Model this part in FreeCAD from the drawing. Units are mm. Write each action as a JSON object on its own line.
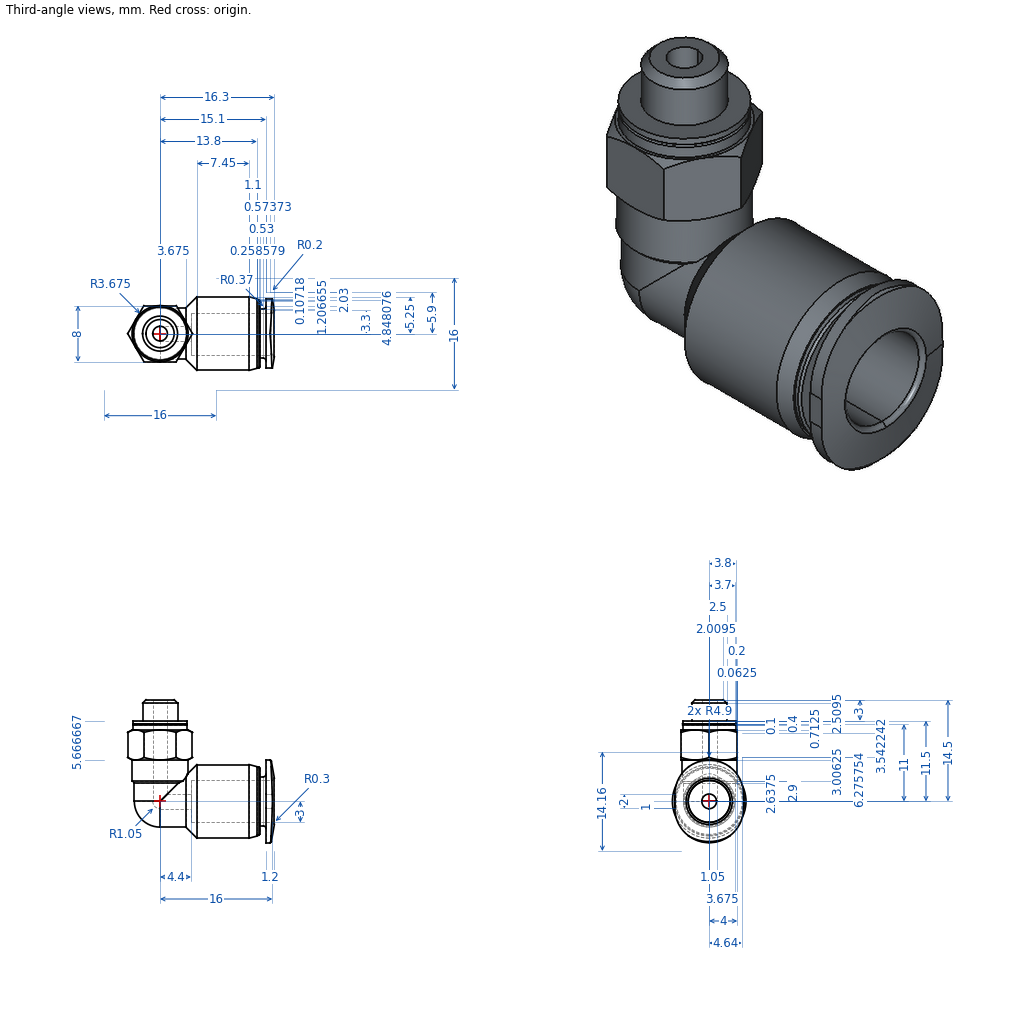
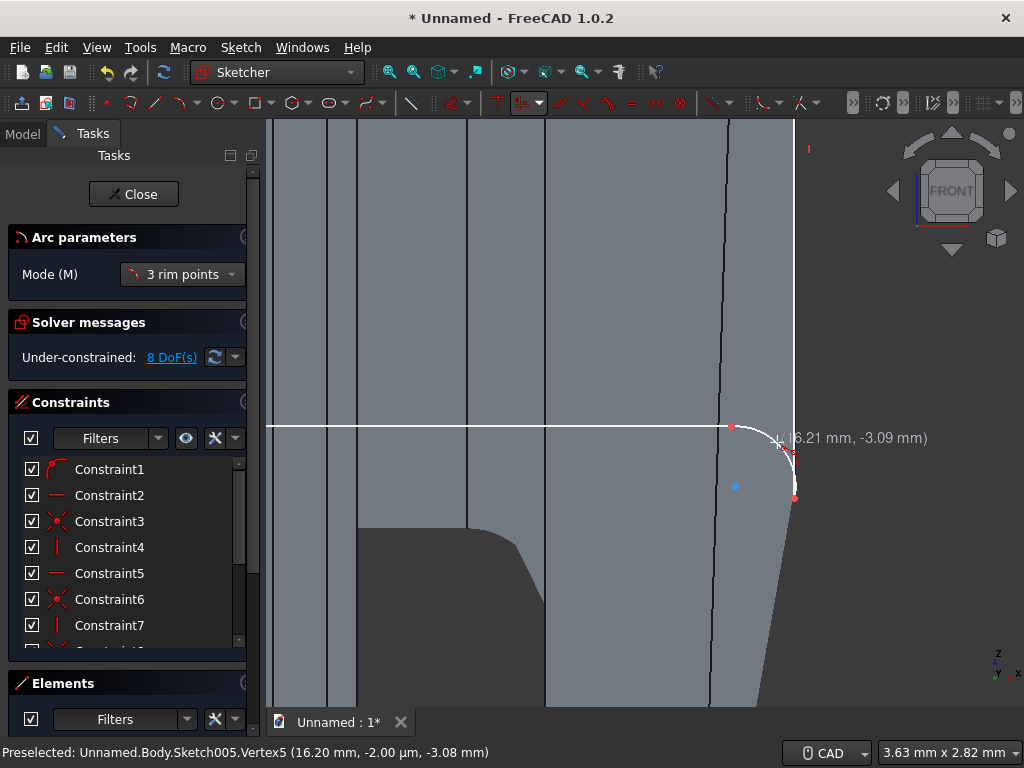
{"action": "scroll", "coordinate": [775, 447], "scroll_direction": "down", "scroll_amount": 11}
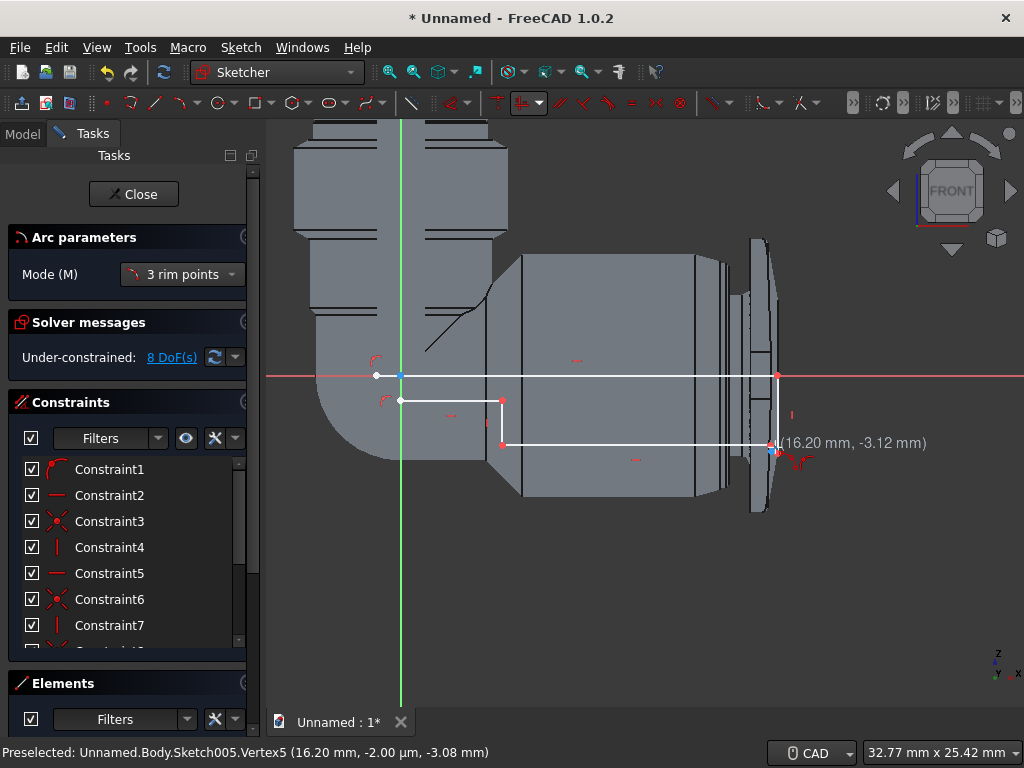
{"action": "left_click", "coordinate": [401, 401]}
{"action": "left_click", "coordinate": [377, 376]}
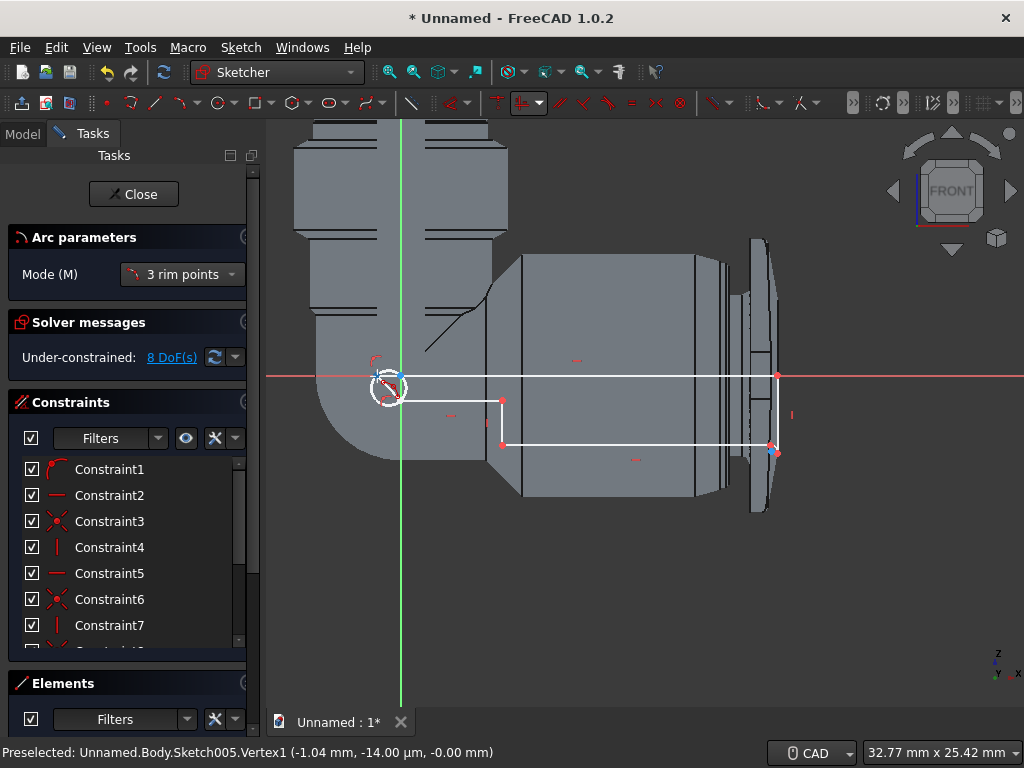
{"action": "scroll", "coordinate": [384, 393], "scroll_direction": "up", "scroll_amount": 5}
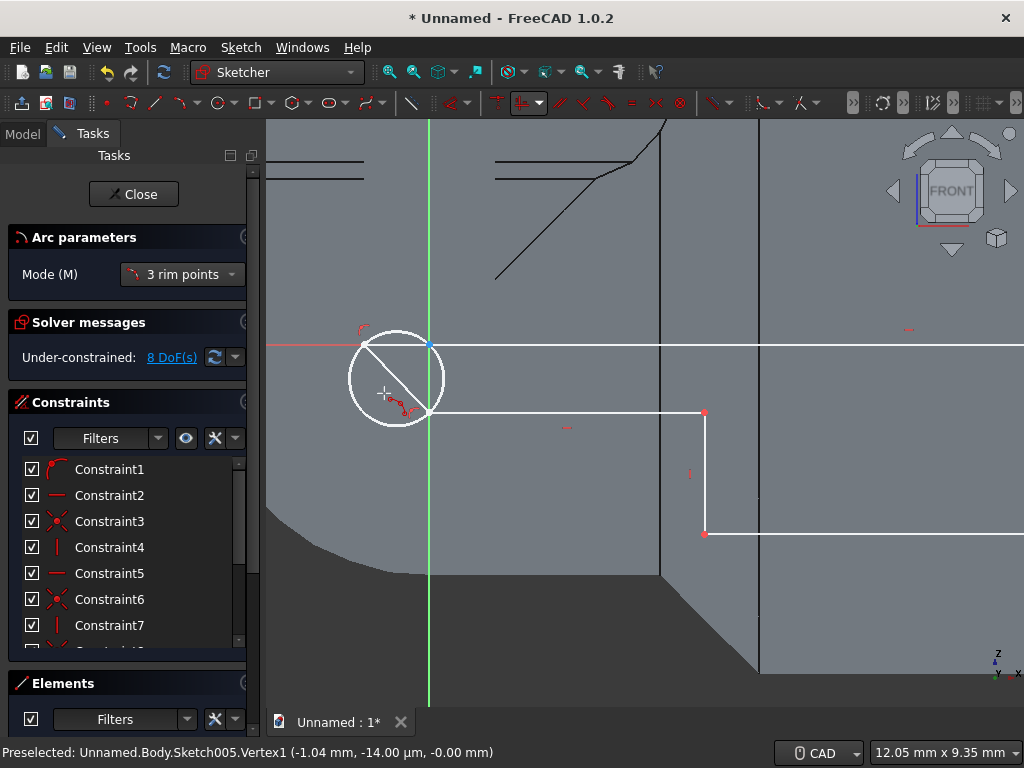
{"action": "left_click", "coordinate": [383, 391]}
{"action": "key", "text": "Escape"}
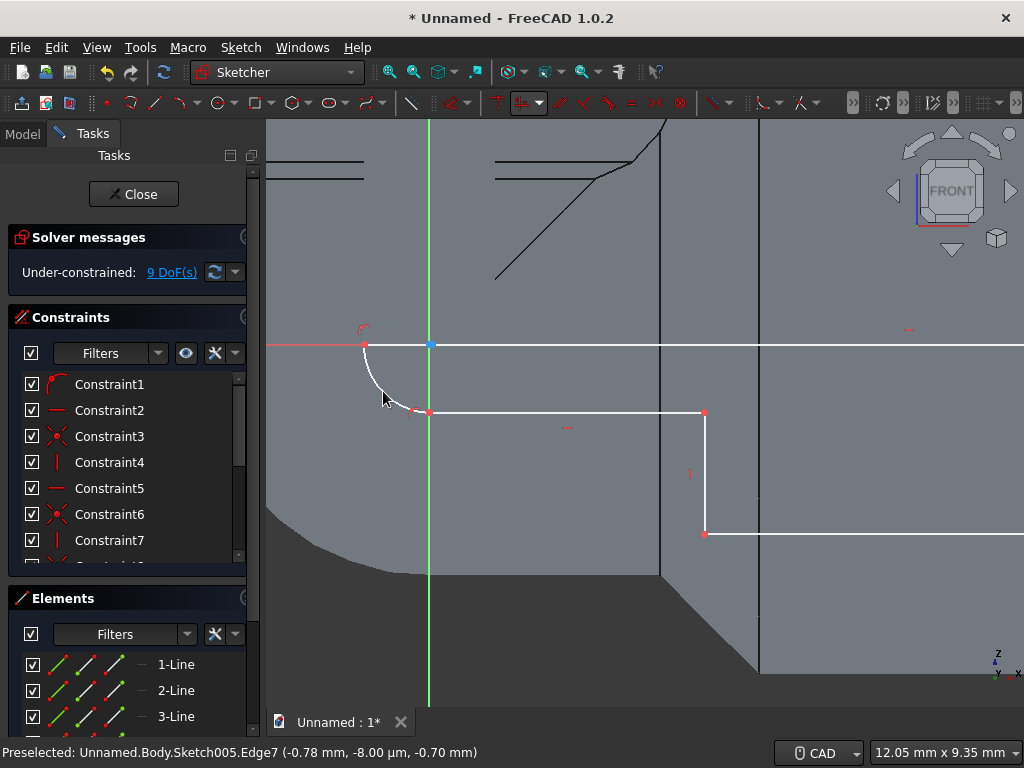
{"action": "scroll", "coordinate": [383, 392], "scroll_direction": "down", "scroll_amount": 5}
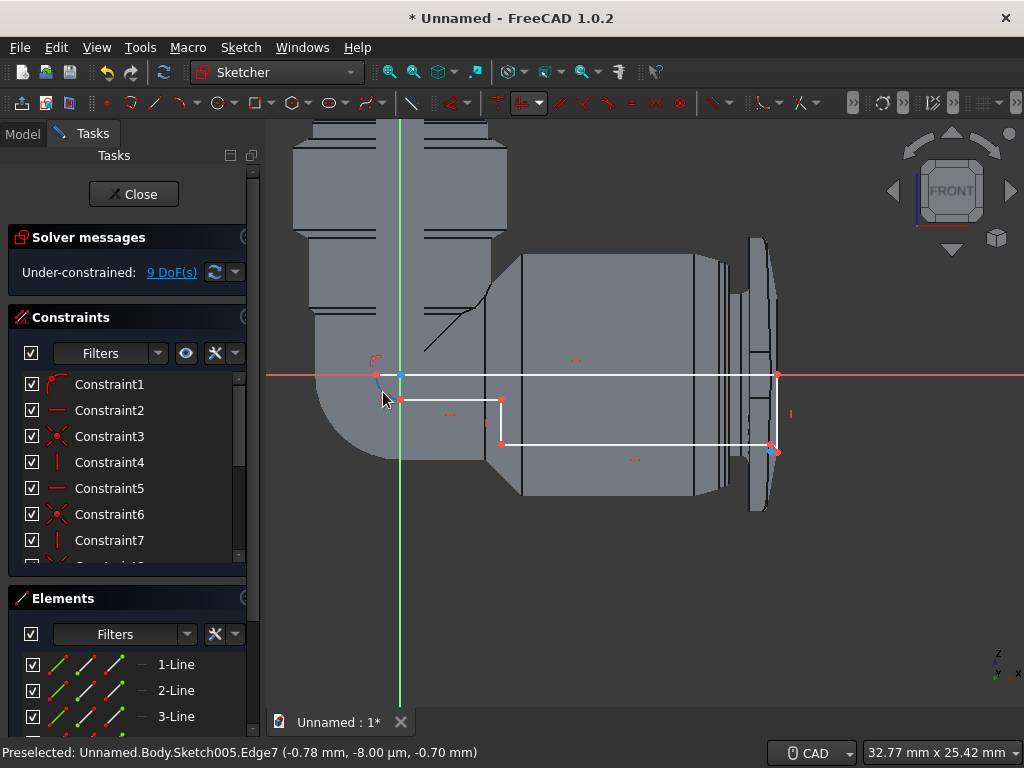
{"action": "left_click", "coordinate": [777, 398]}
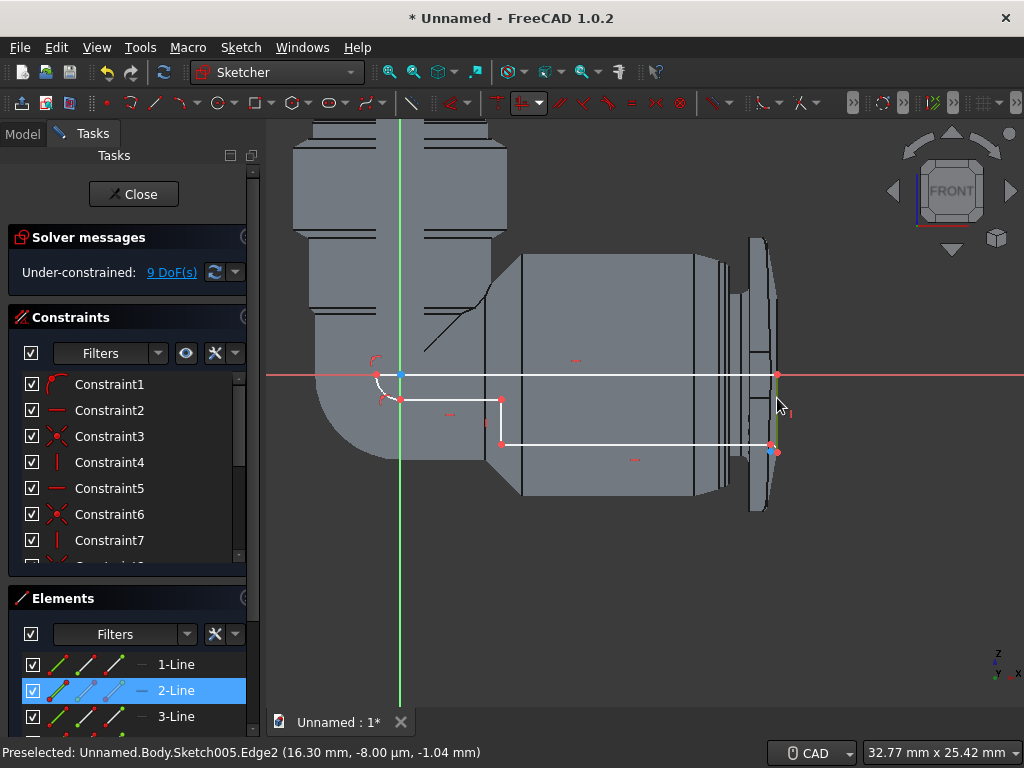
{"action": "scroll", "coordinate": [774, 445], "scroll_direction": "up", "scroll_amount": 8}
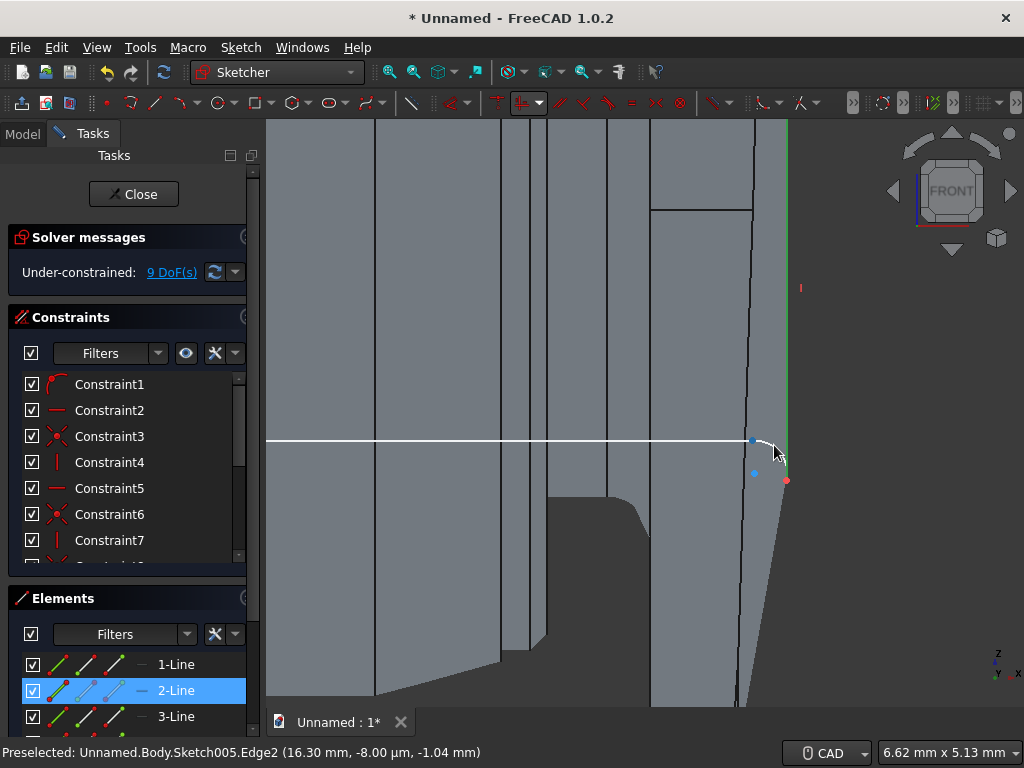
{"action": "left_click", "coordinate": [770, 445]}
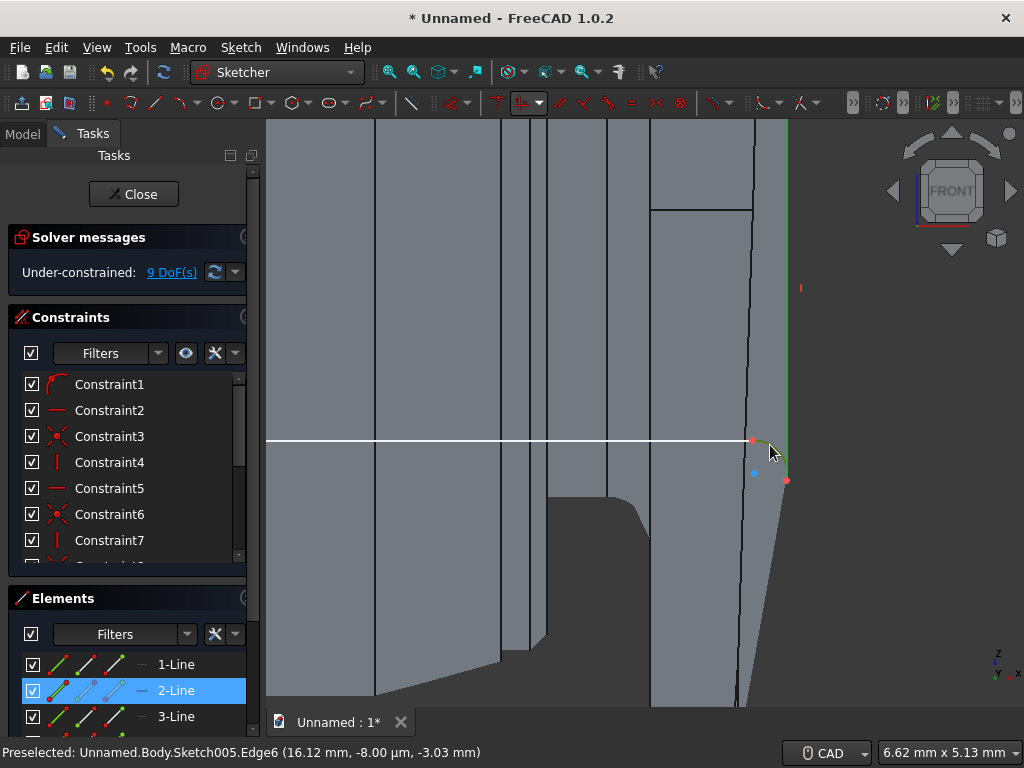
{"action": "left_click", "coordinate": [608, 104]}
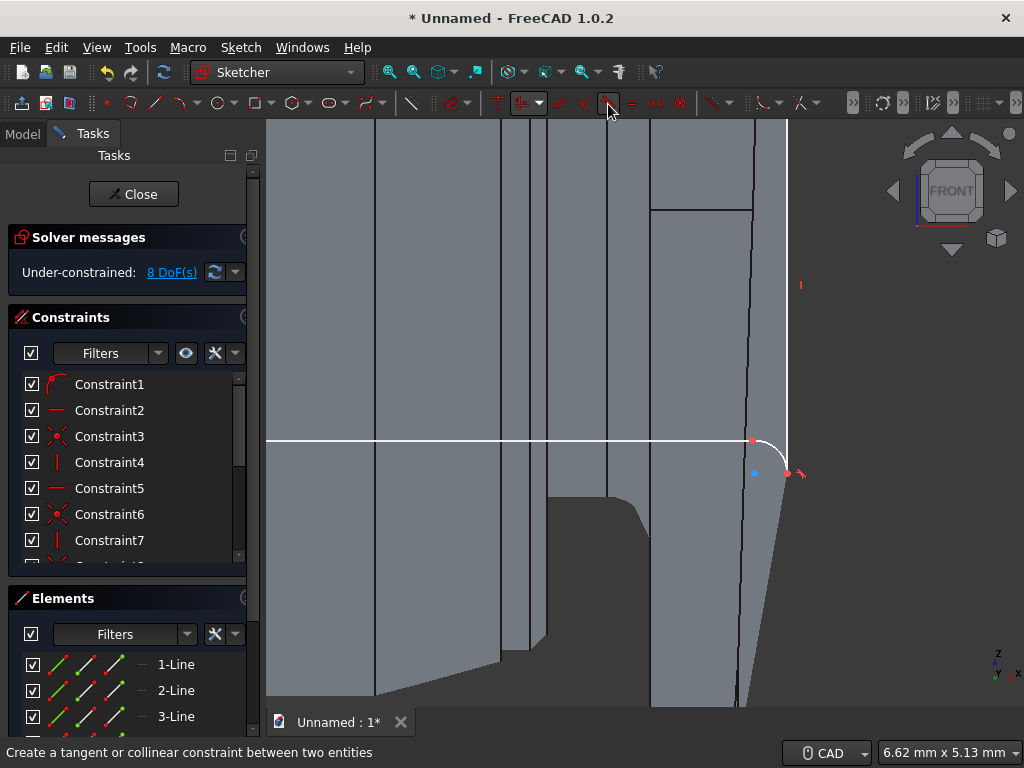
{"action": "scroll", "coordinate": [775, 445], "scroll_direction": "down", "scroll_amount": 8}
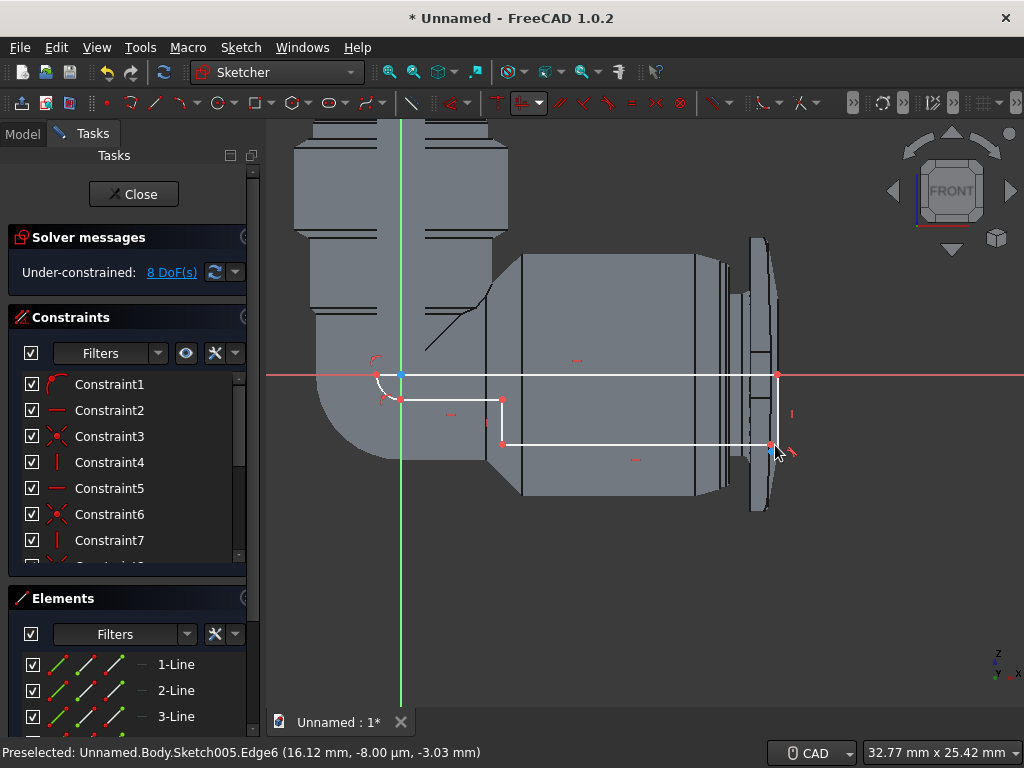
{"action": "left_click", "coordinate": [690, 445]}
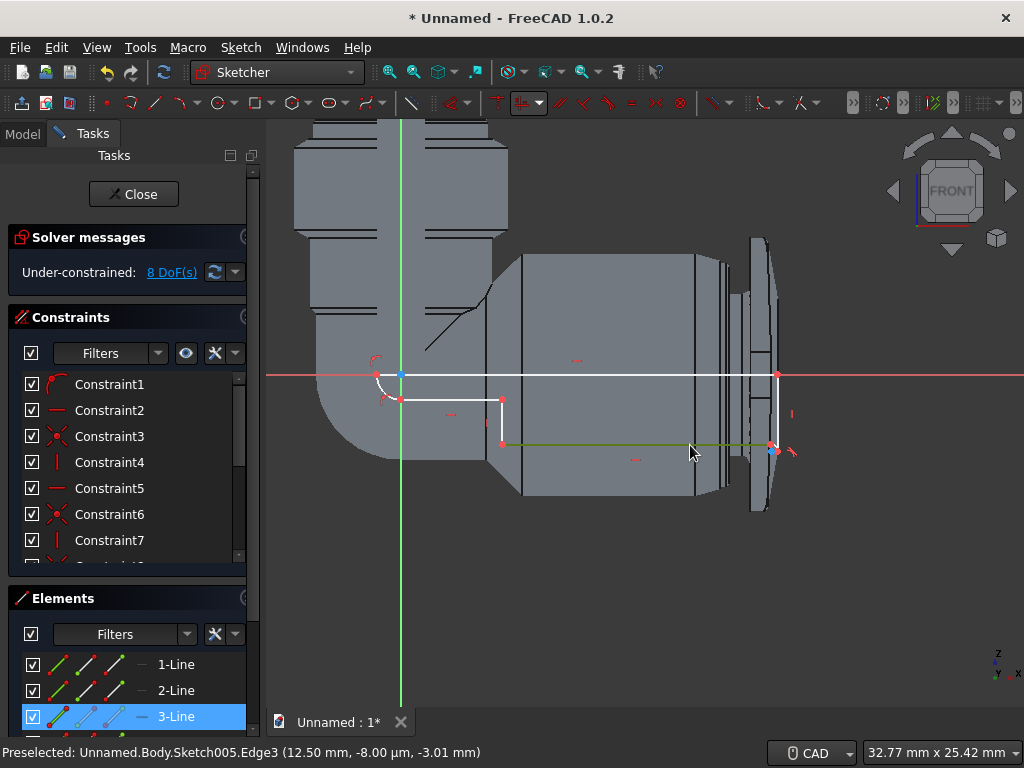
{"action": "scroll", "coordinate": [774, 445], "scroll_direction": "up", "scroll_amount": 8}